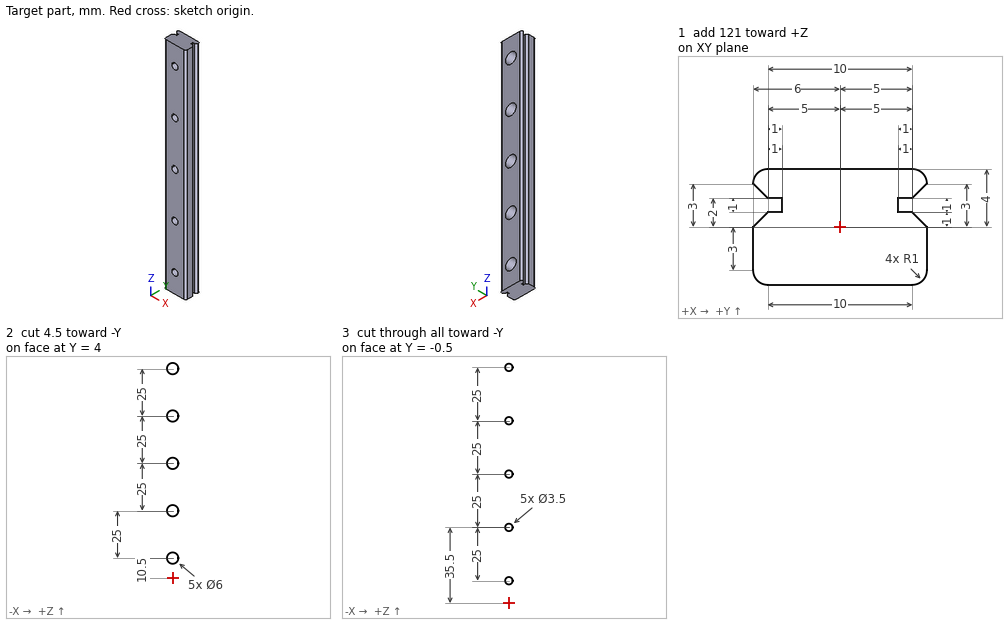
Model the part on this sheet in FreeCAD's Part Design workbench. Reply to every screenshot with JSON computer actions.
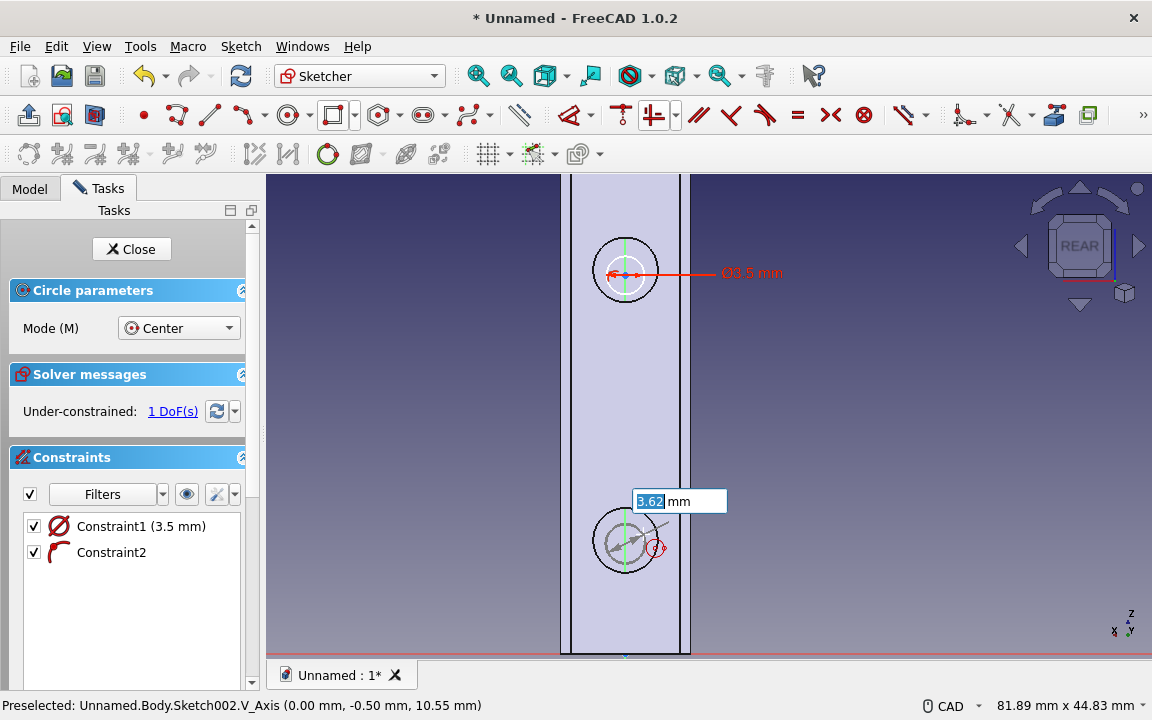
{"action": "type", "text": "3.5"}
{"action": "key", "text": "Return"}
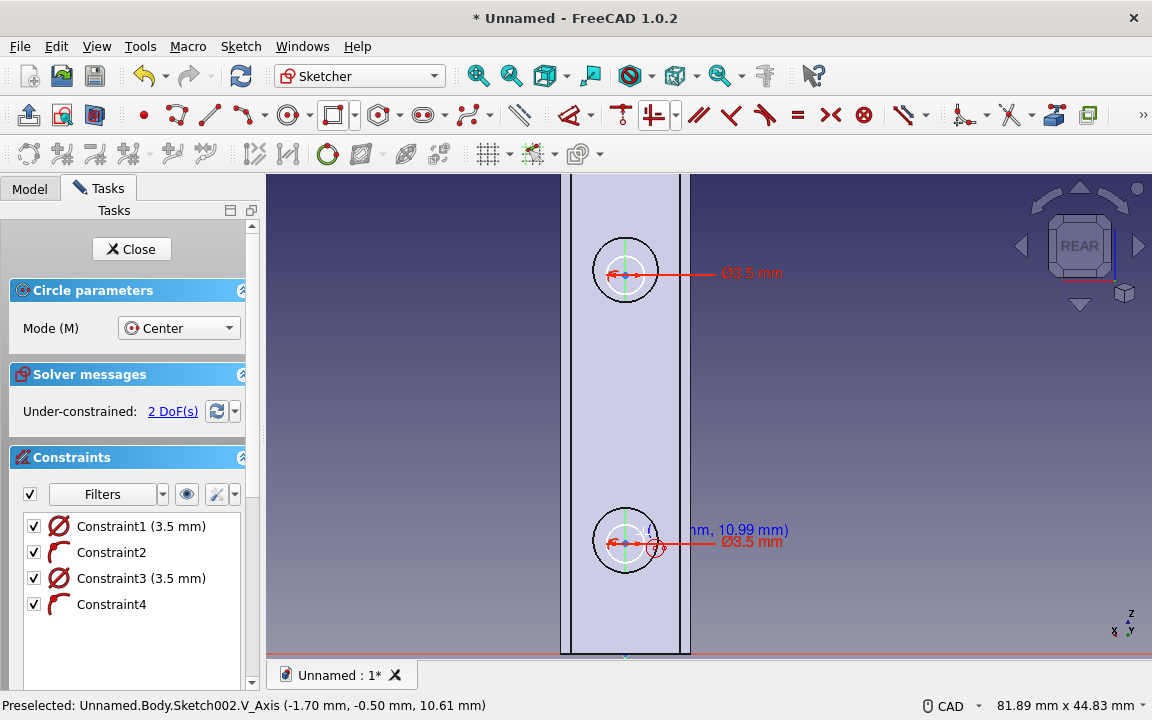
{"action": "scroll", "coordinate": [645, 538], "scroll_direction": "down", "scroll_amount": 7}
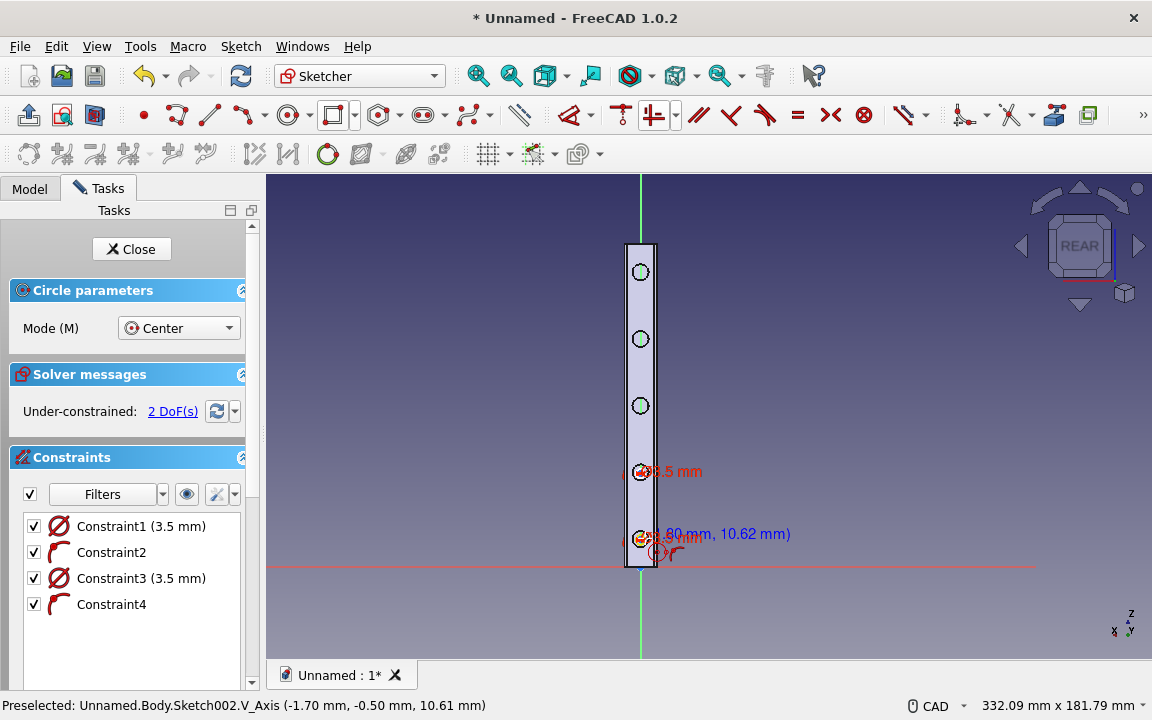
{"action": "scroll", "coordinate": [641, 406], "scroll_direction": "up", "scroll_amount": 8}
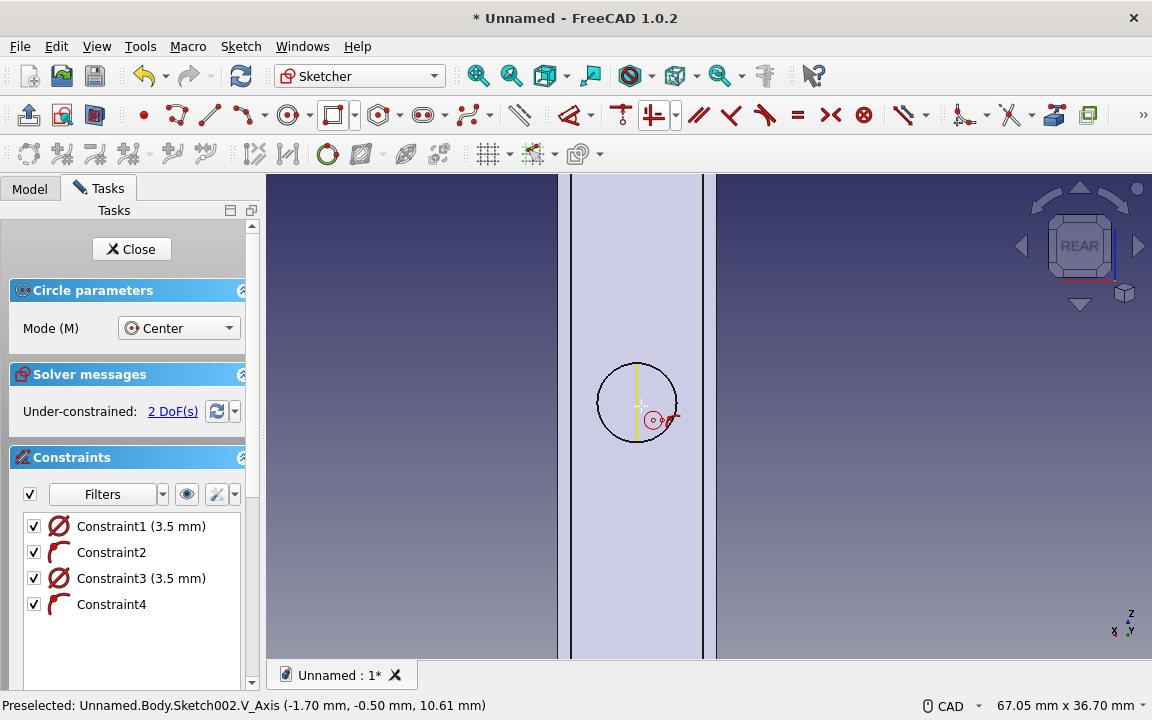
{"action": "scroll", "coordinate": [641, 405], "scroll_direction": "down", "scroll_amount": 8}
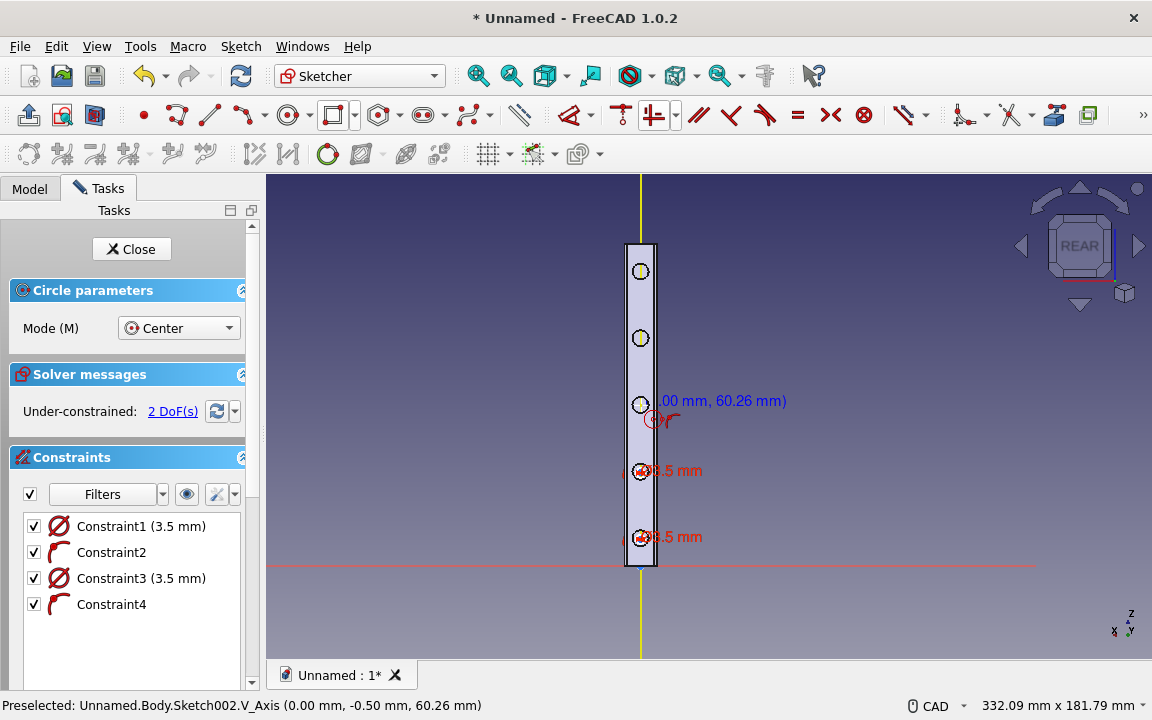
{"action": "left_click", "coordinate": [641, 405]}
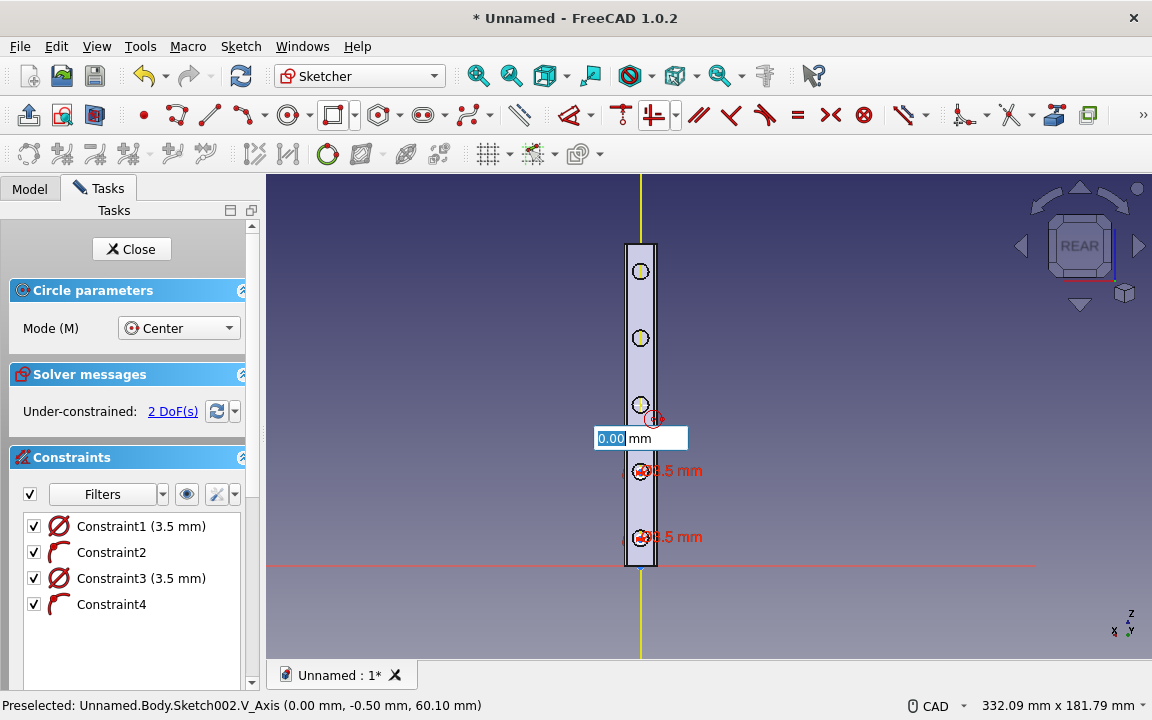
{"action": "scroll", "coordinate": [645, 403], "scroll_direction": "up", "scroll_amount": 7}
{"action": "mouse_move", "coordinate": [643, 403]}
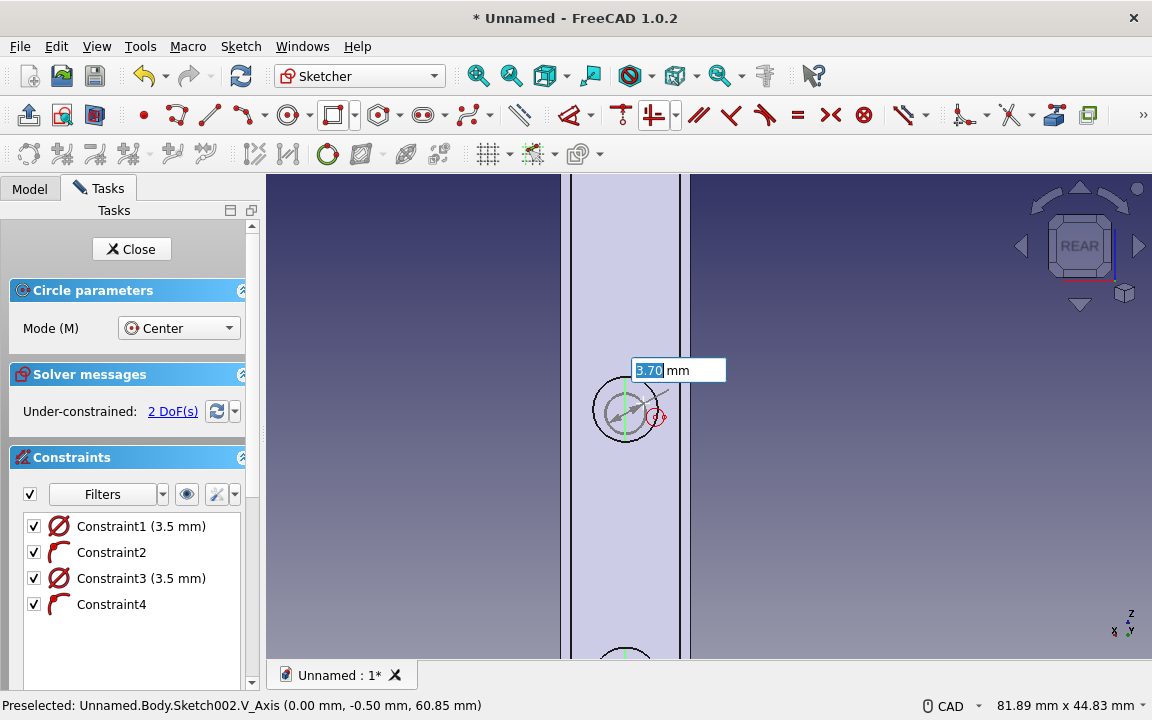
{"action": "type", "text": "3.5"}
{"action": "key", "text": "Return"}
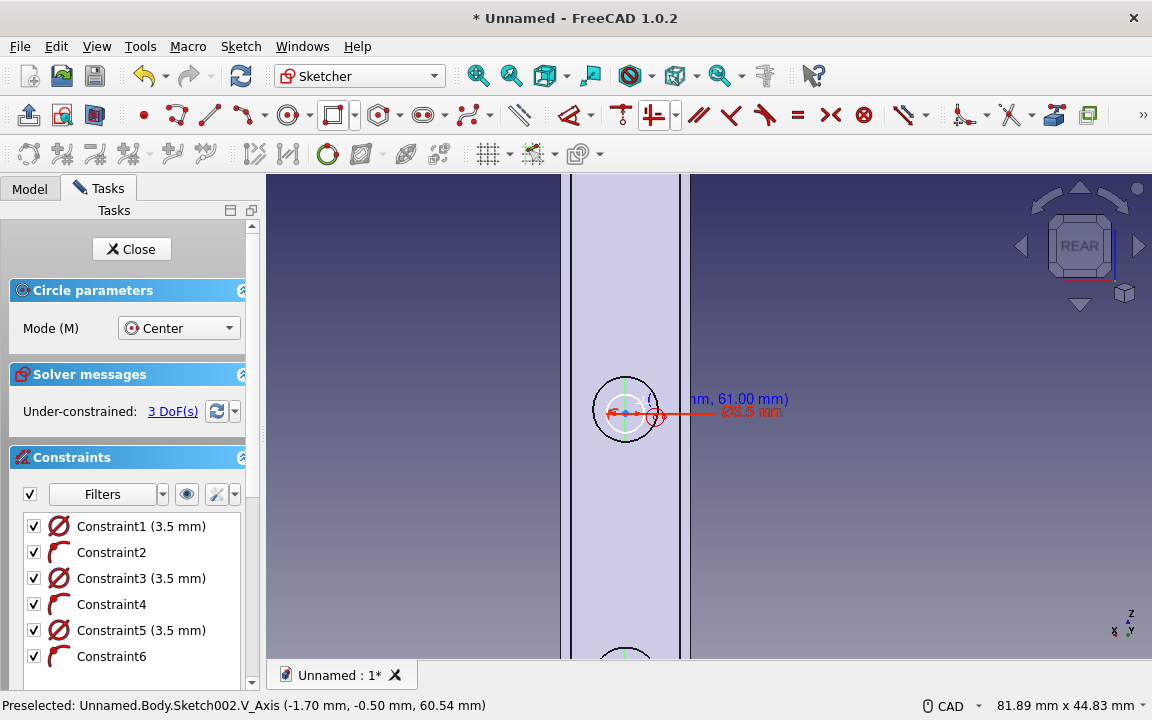
{"action": "scroll", "coordinate": [645, 403], "scroll_direction": "down", "scroll_amount": 7}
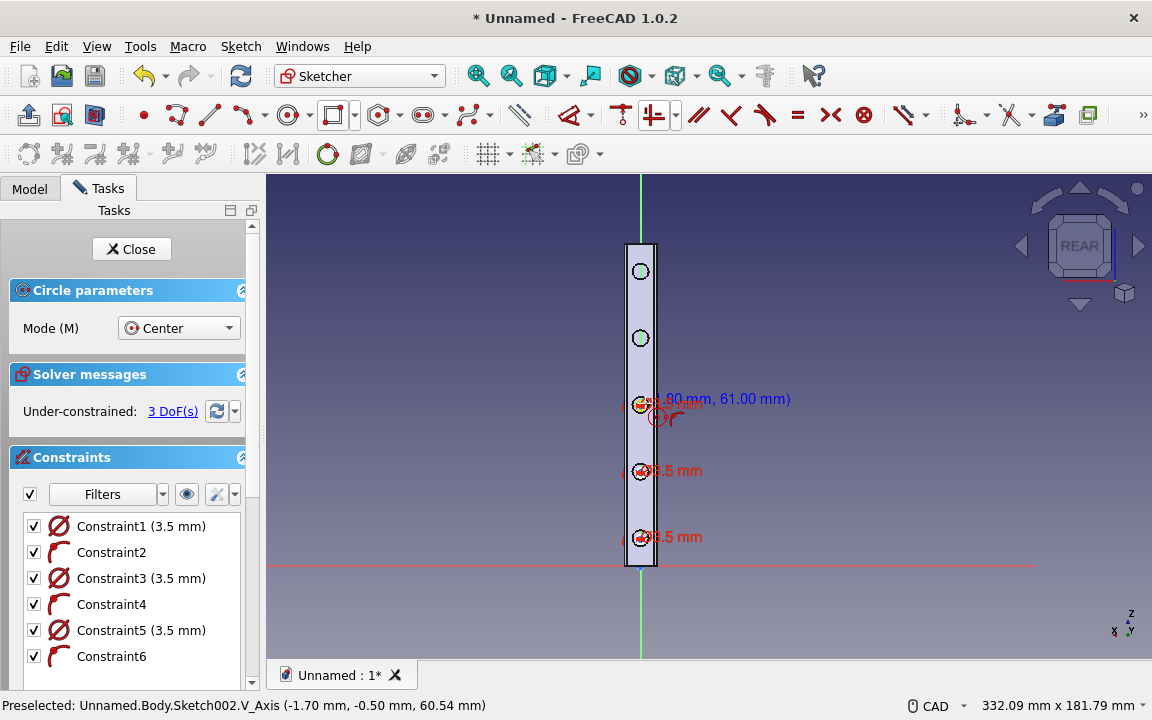
{"action": "scroll", "coordinate": [641, 338], "scroll_direction": "up", "scroll_amount": 8}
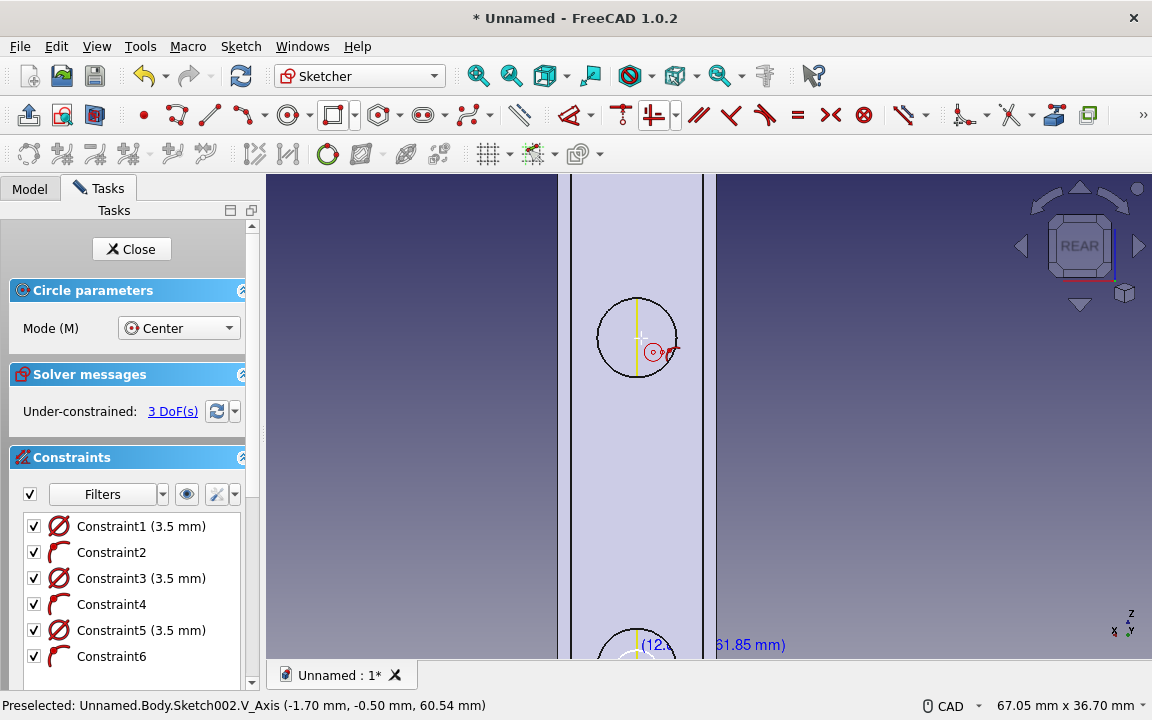
{"action": "scroll", "coordinate": [641, 338], "scroll_direction": "down", "scroll_amount": 8}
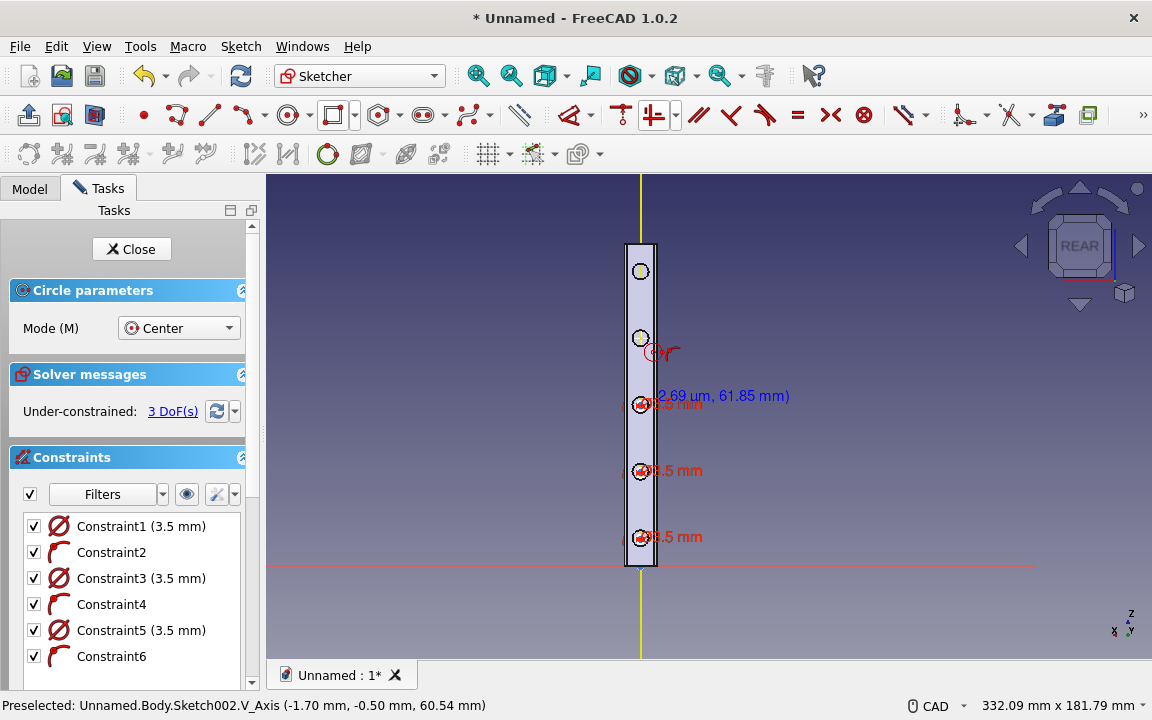
{"action": "left_click", "coordinate": [641, 338]}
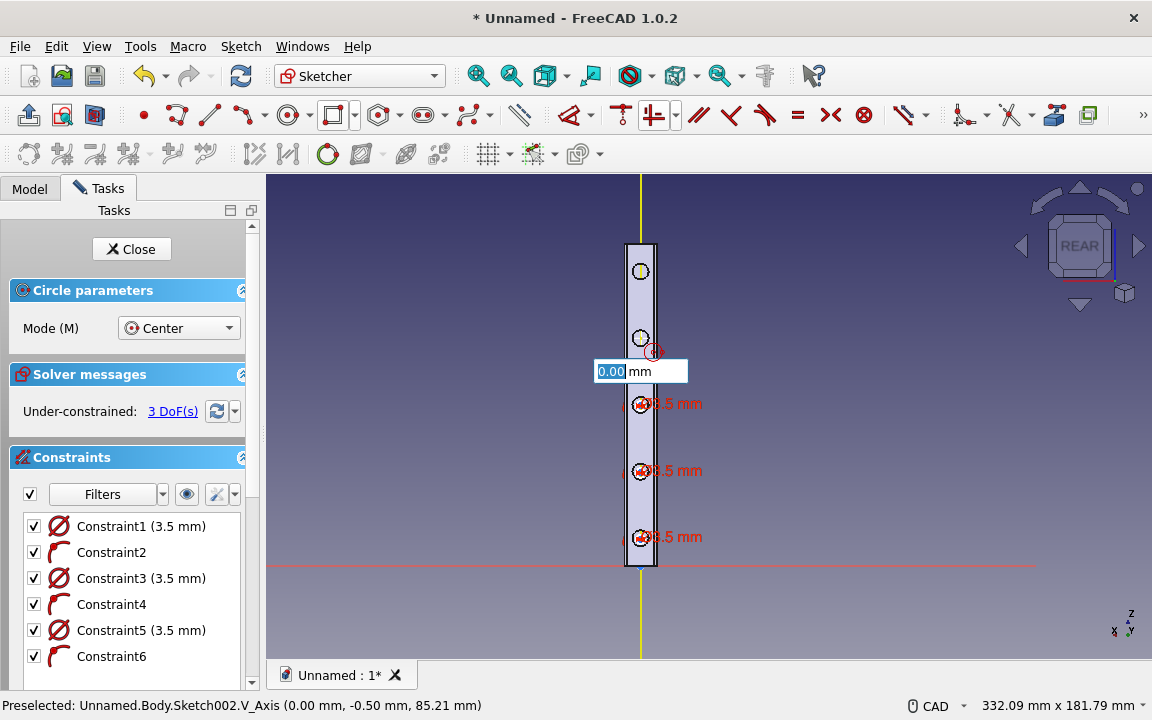
{"action": "scroll", "coordinate": [645, 337], "scroll_direction": "up", "scroll_amount": 7}
{"action": "mouse_move", "coordinate": [643, 335]}